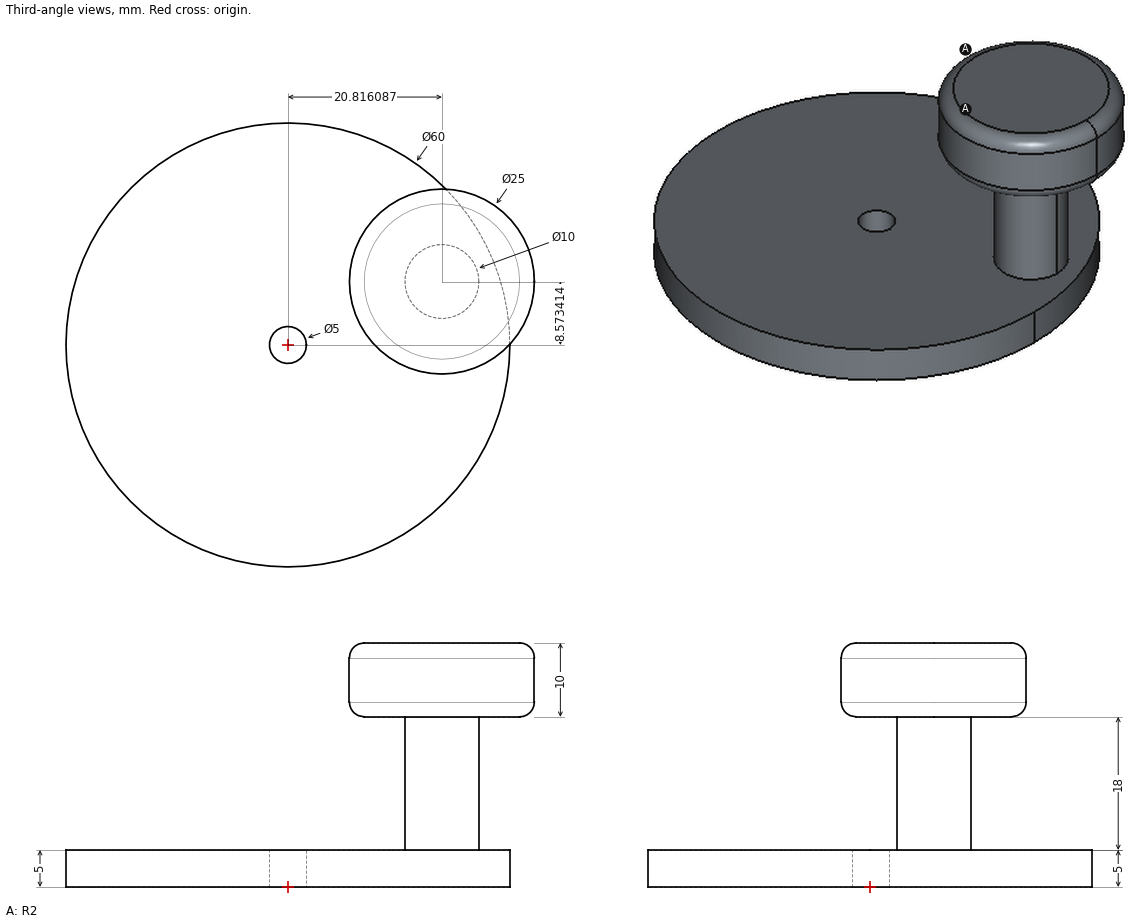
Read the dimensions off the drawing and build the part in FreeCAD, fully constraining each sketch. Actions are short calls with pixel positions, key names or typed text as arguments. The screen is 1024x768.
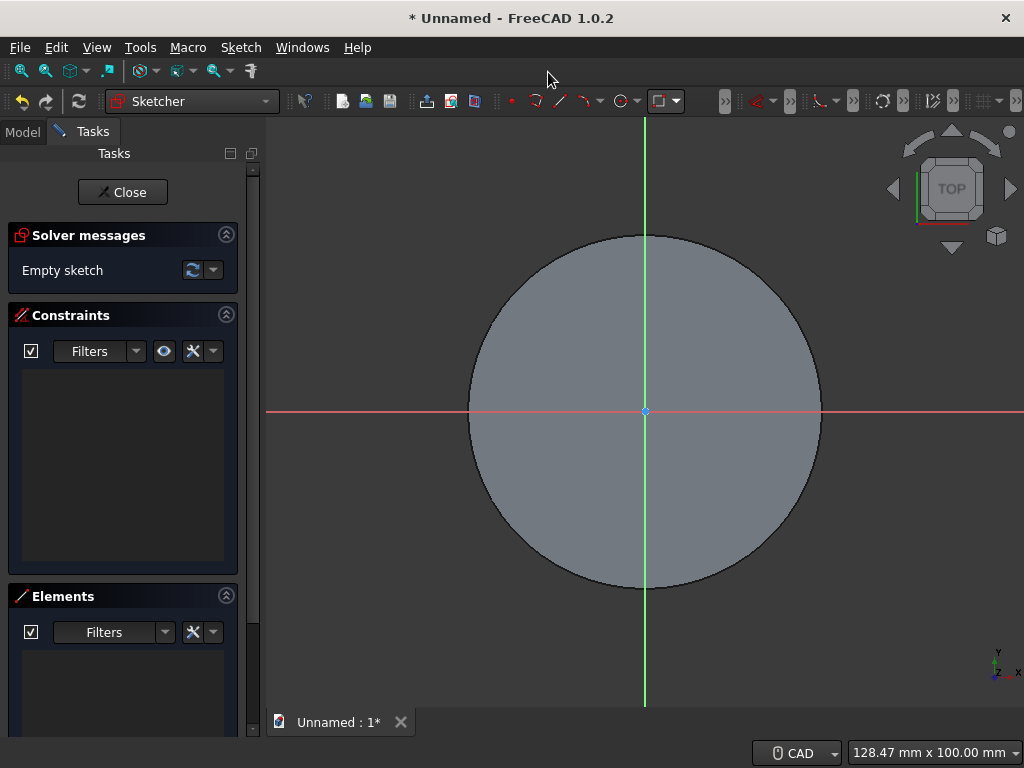
scroll(650, 412, up, 13)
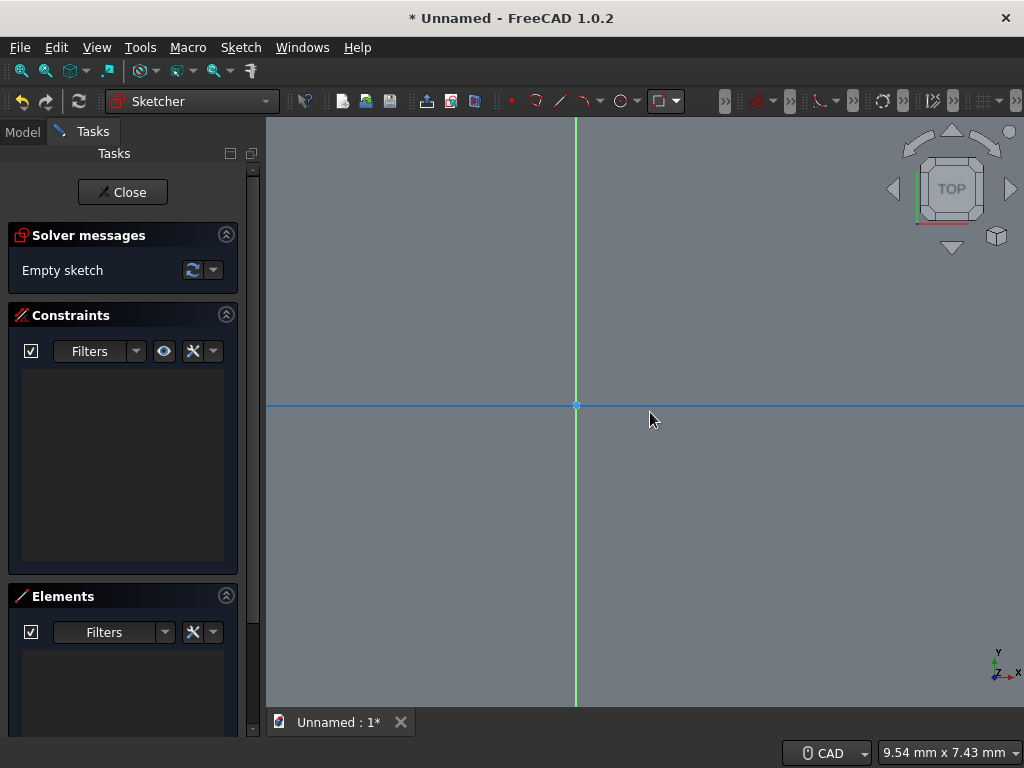
click(622, 102)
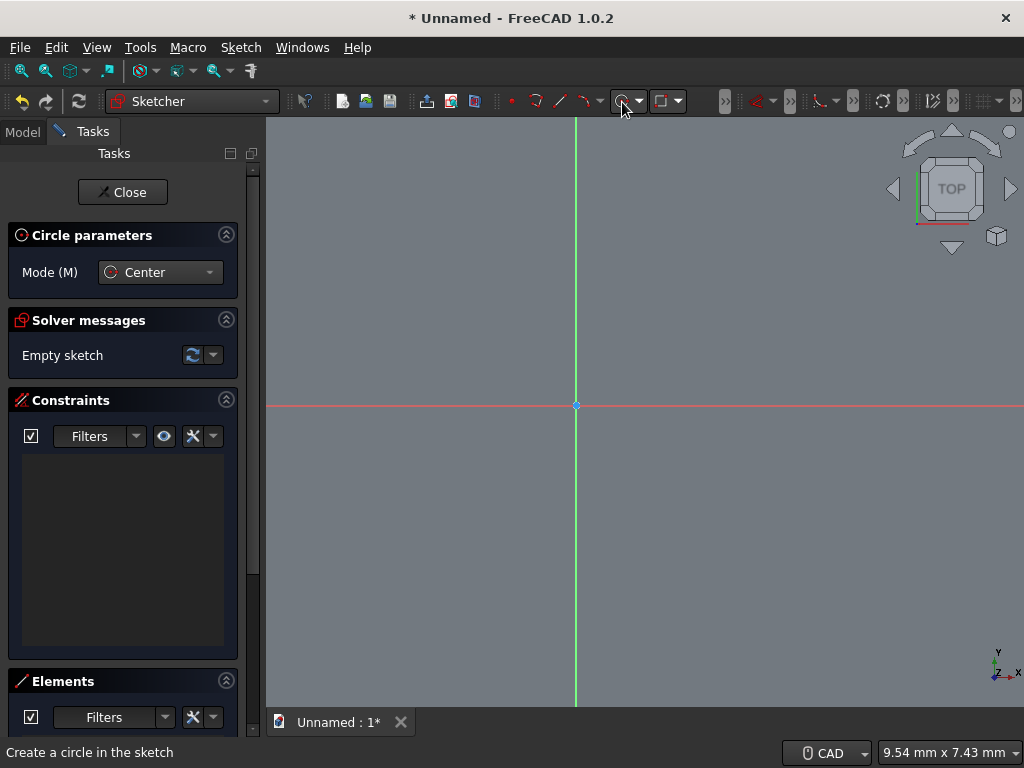
click(576, 406)
move(717, 265)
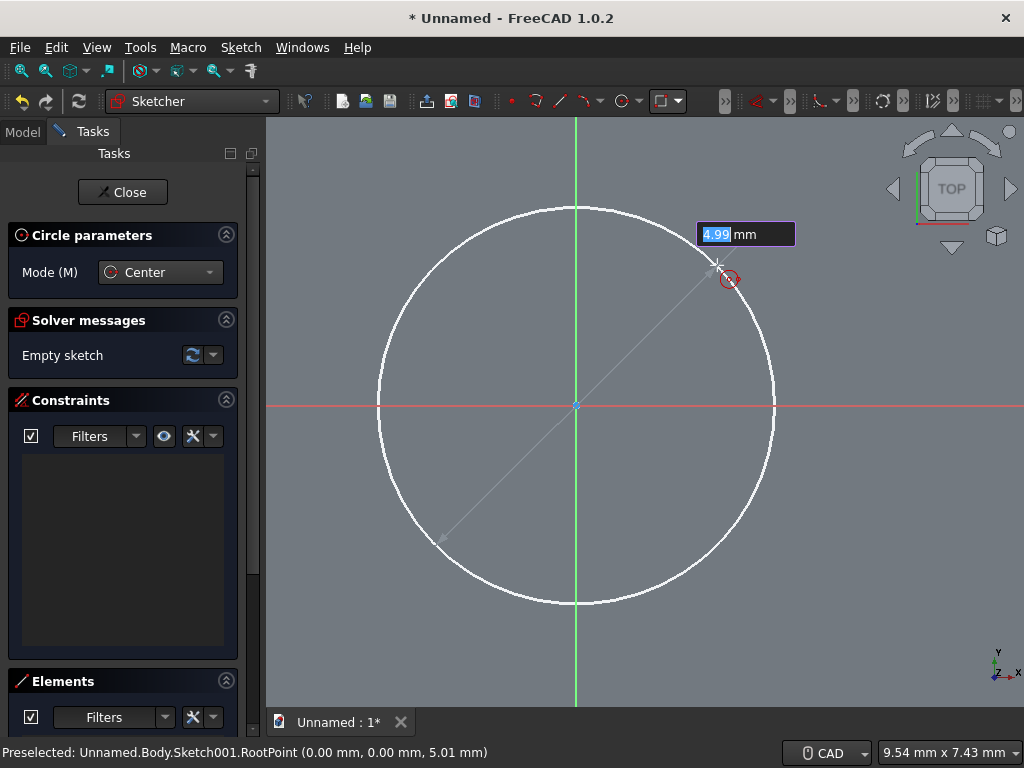
text(5)
key(Return)
key(Escape)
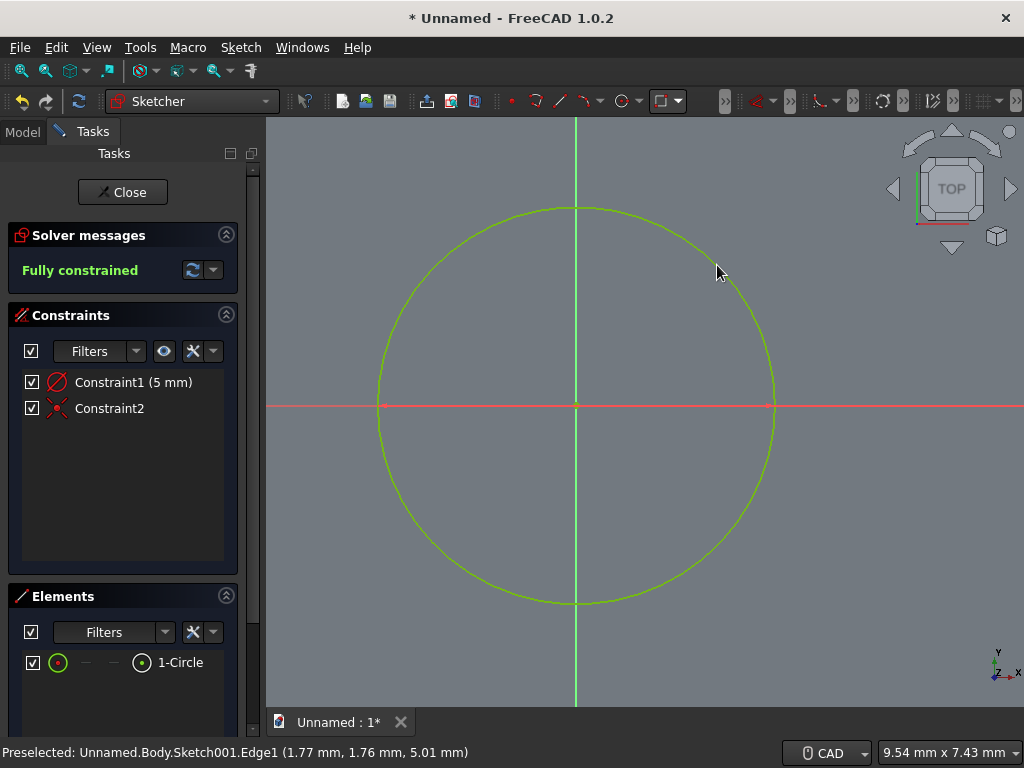
click(123, 192)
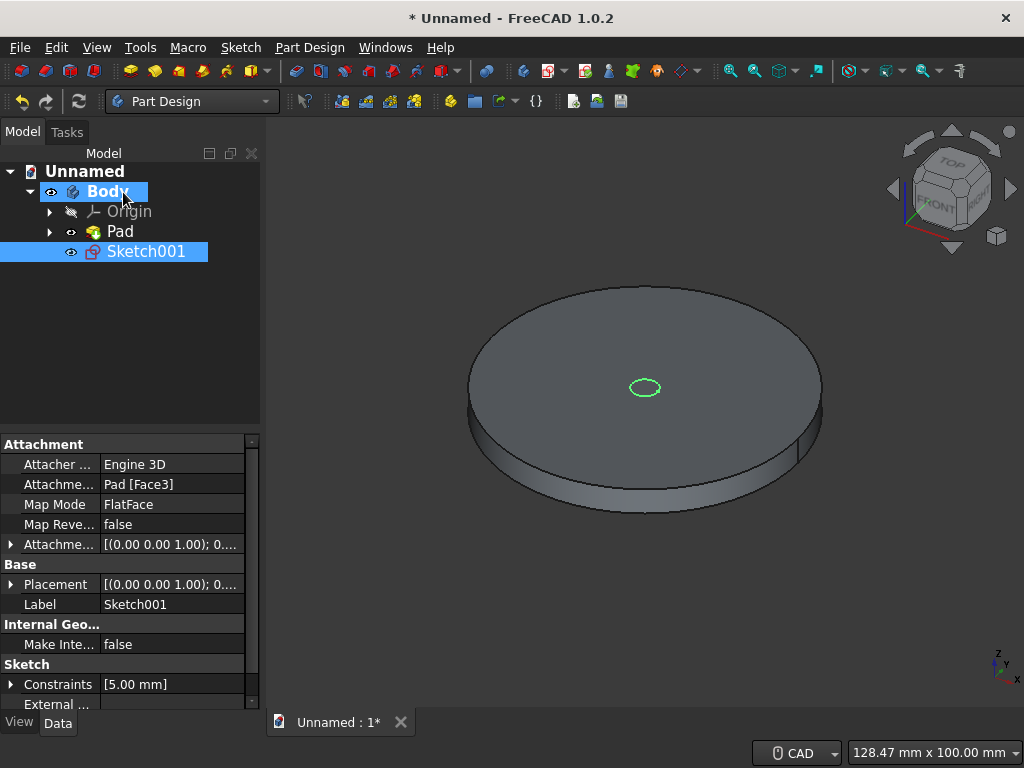
click(298, 72)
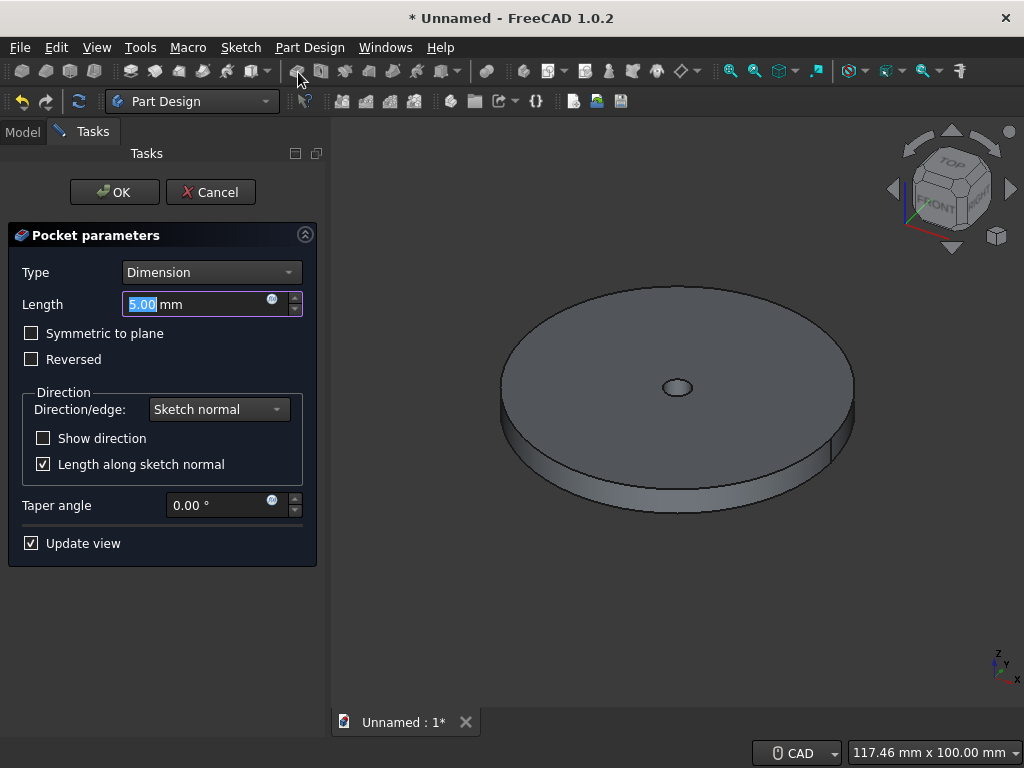
text(5)
key(Tab)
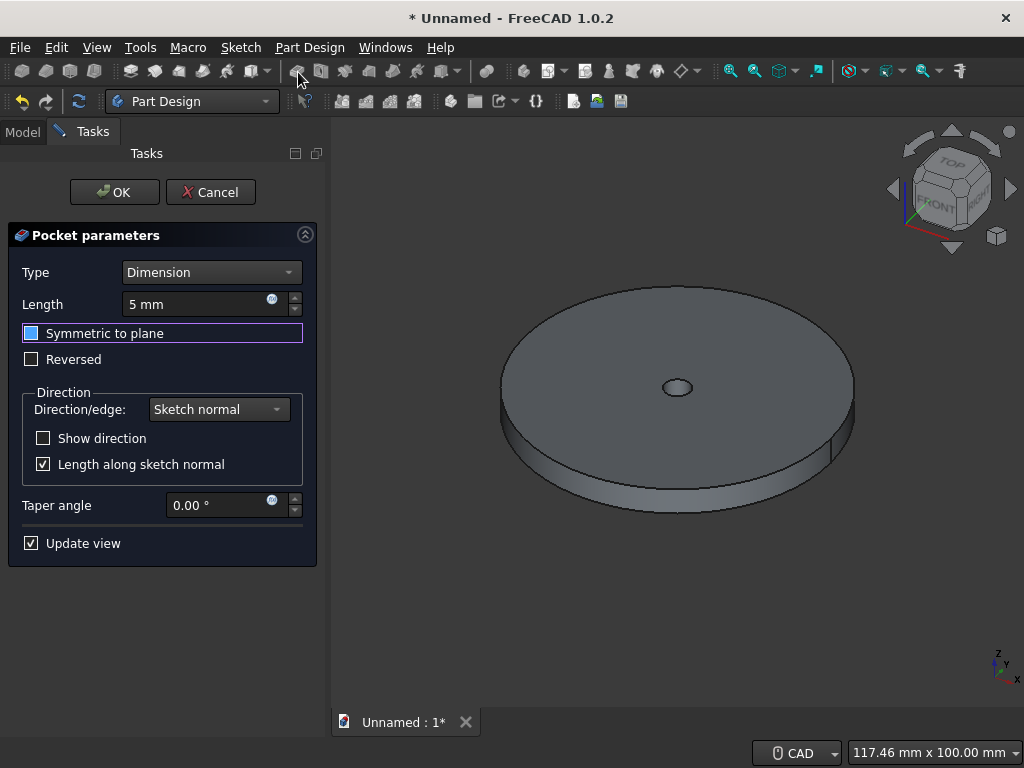
click(115, 192)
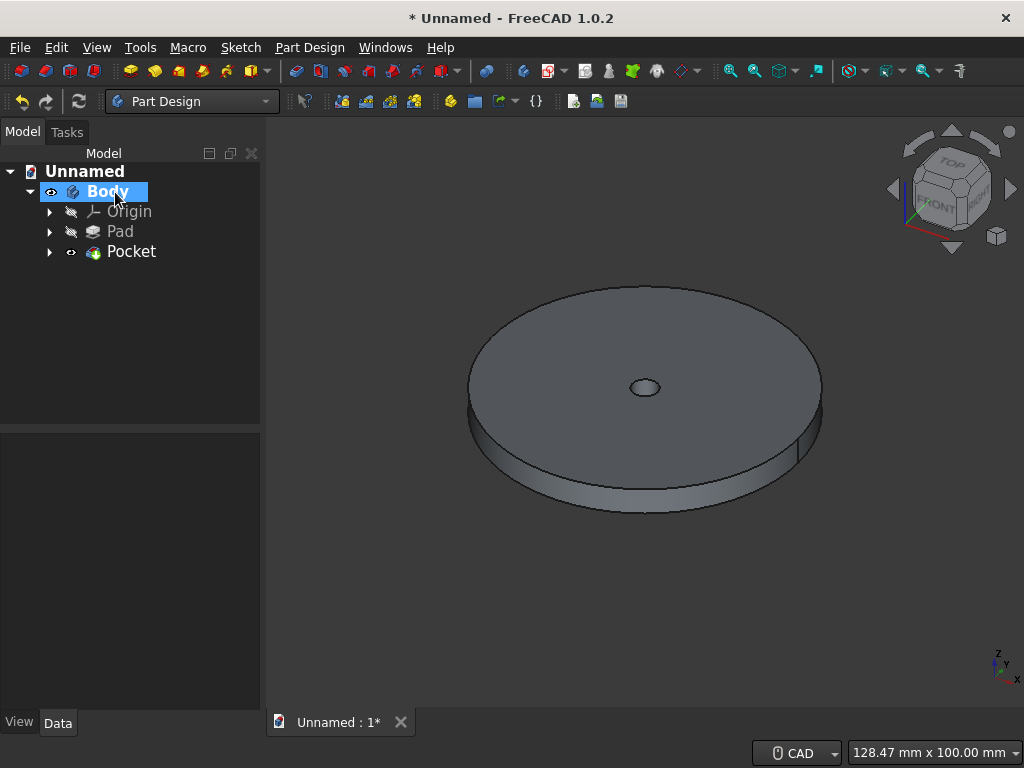
click(594, 437)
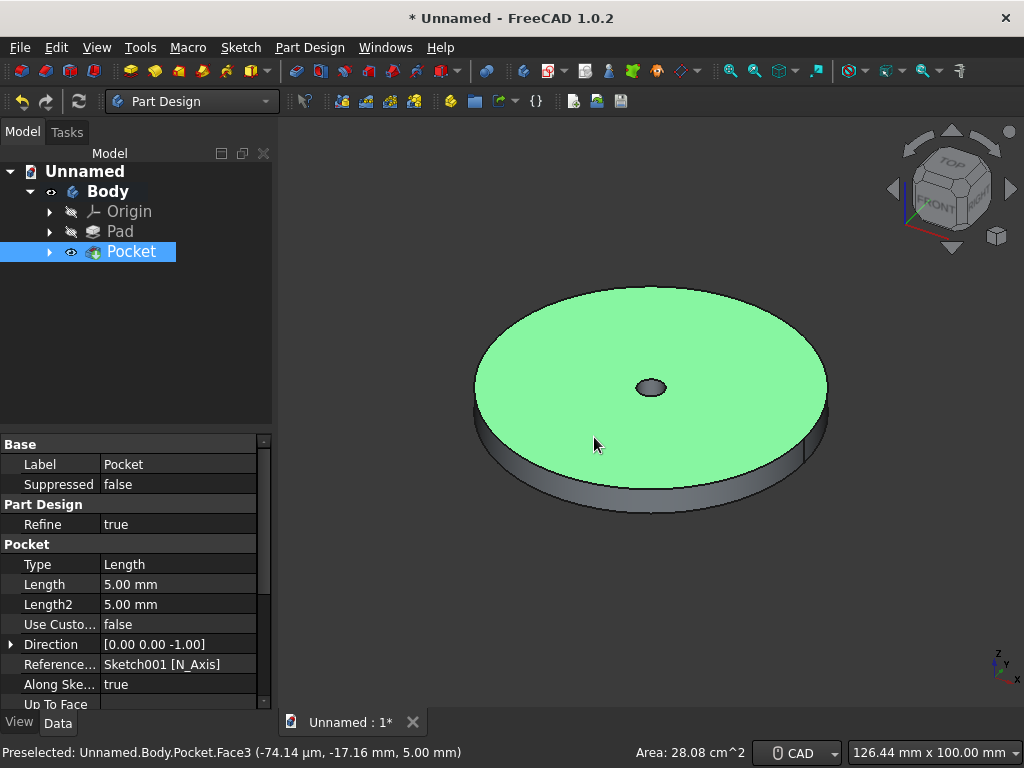
click(548, 72)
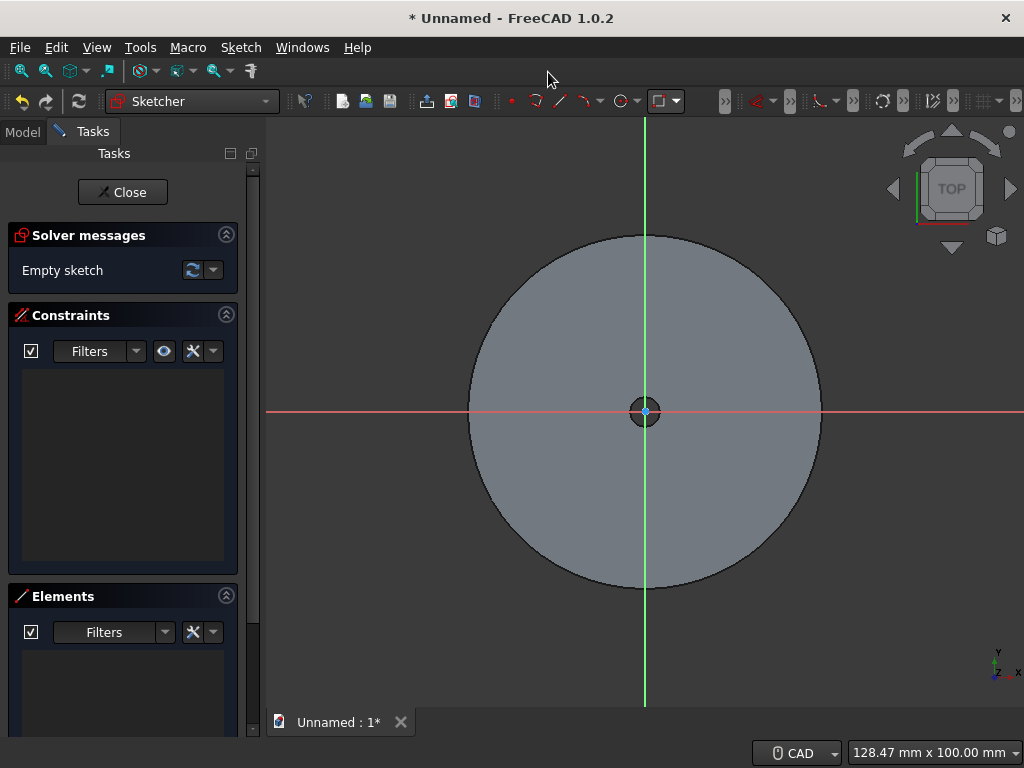
scroll(806, 351, up, 9)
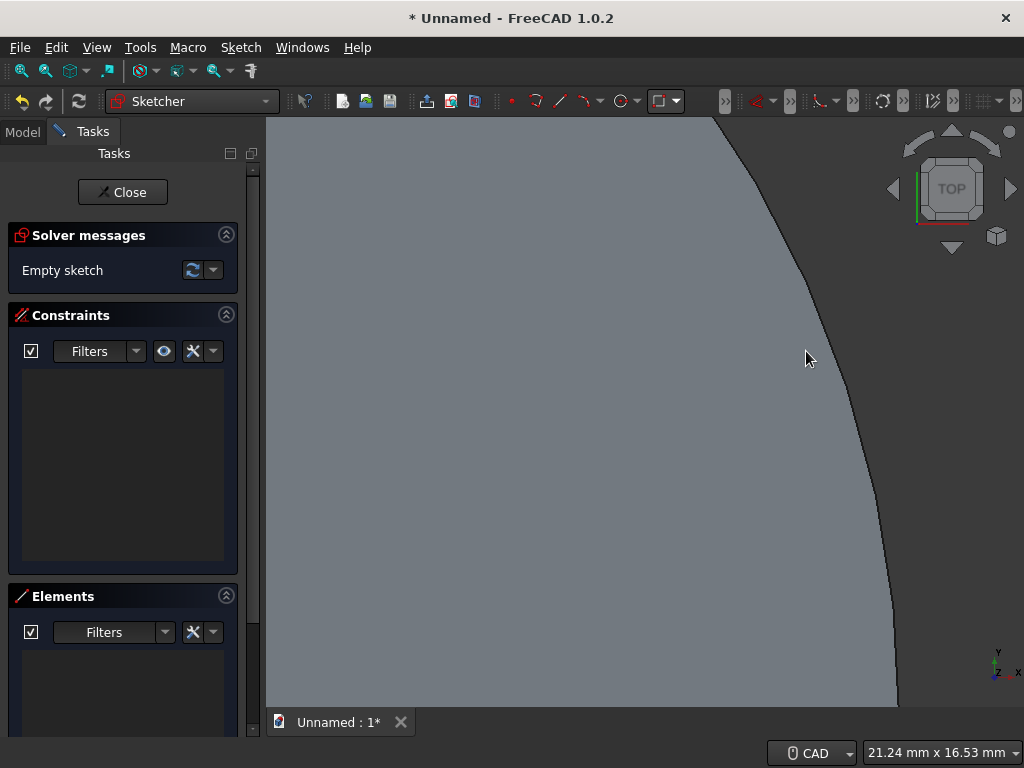
click(622, 102)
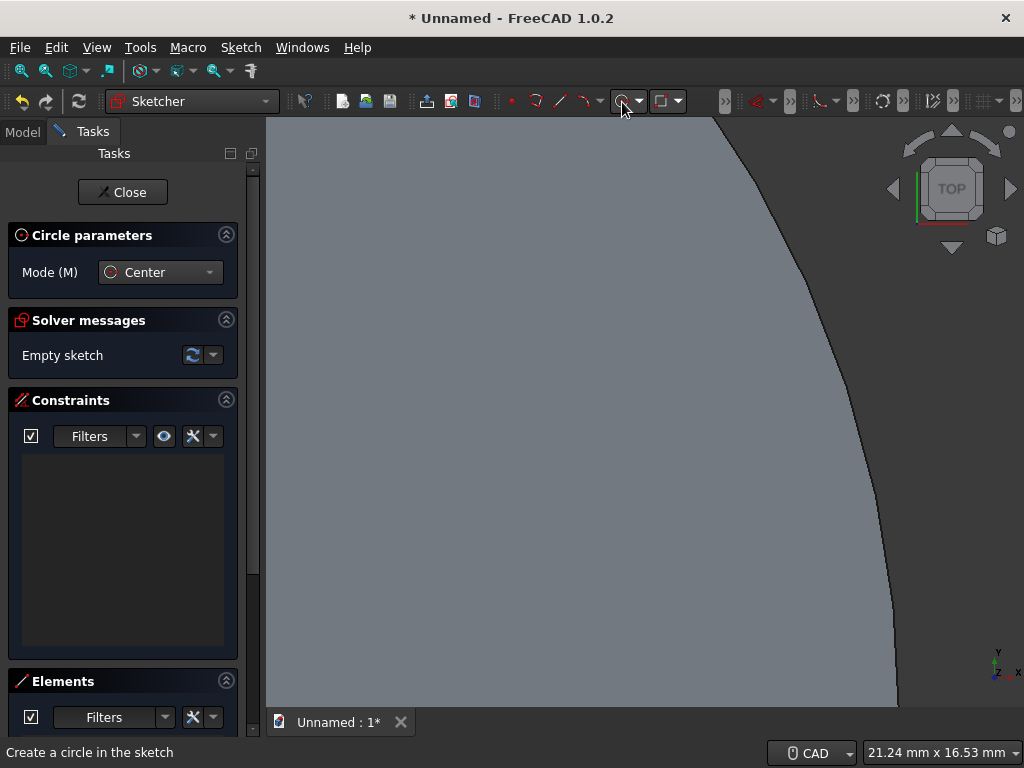
click(571, 412)
move(698, 286)